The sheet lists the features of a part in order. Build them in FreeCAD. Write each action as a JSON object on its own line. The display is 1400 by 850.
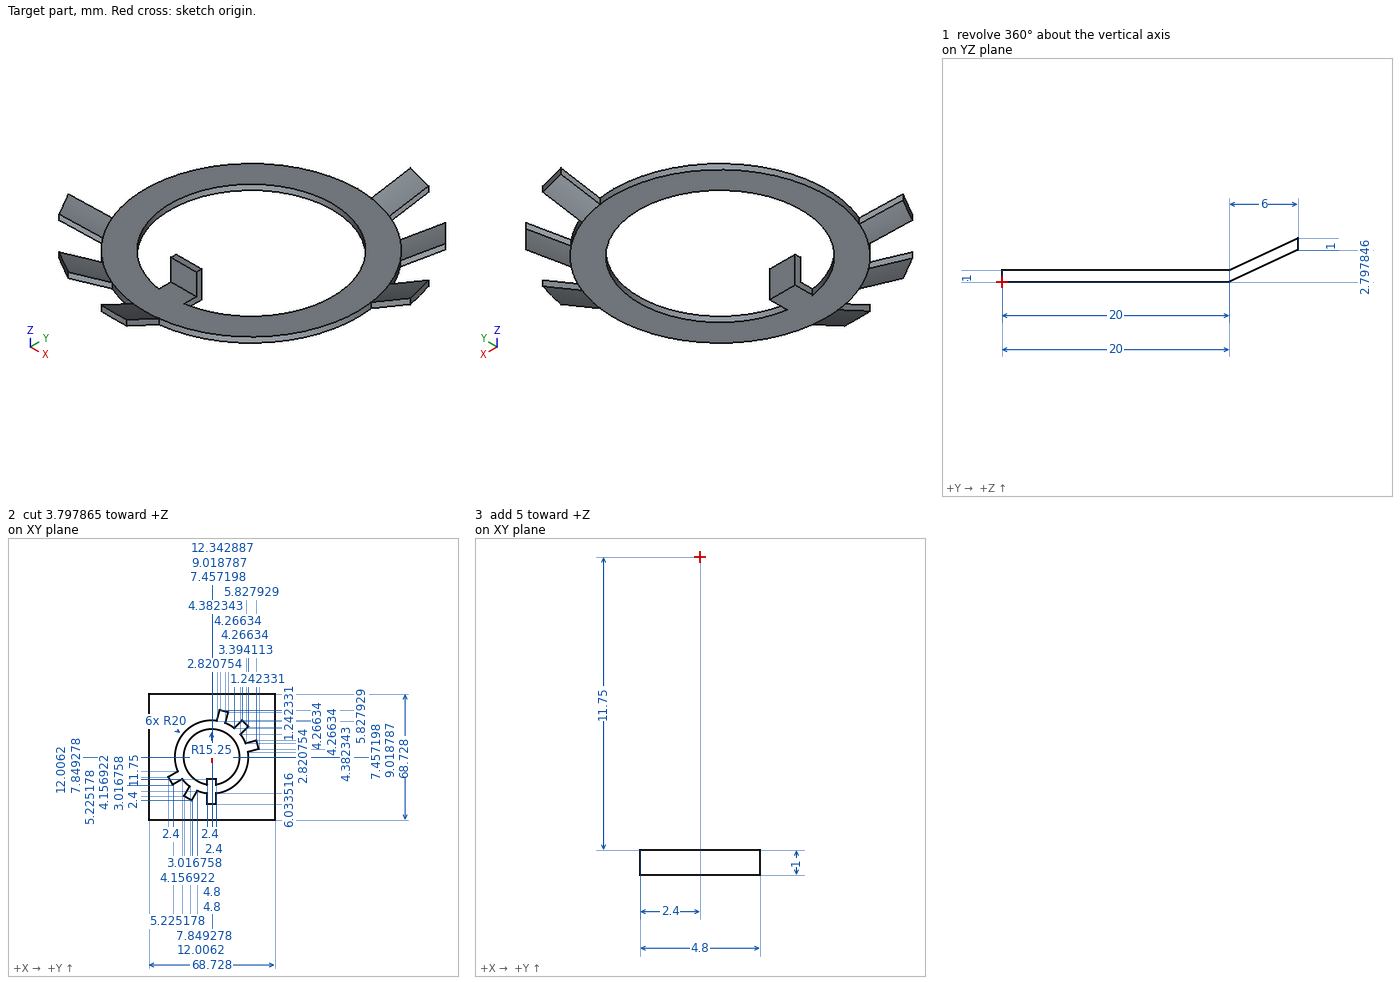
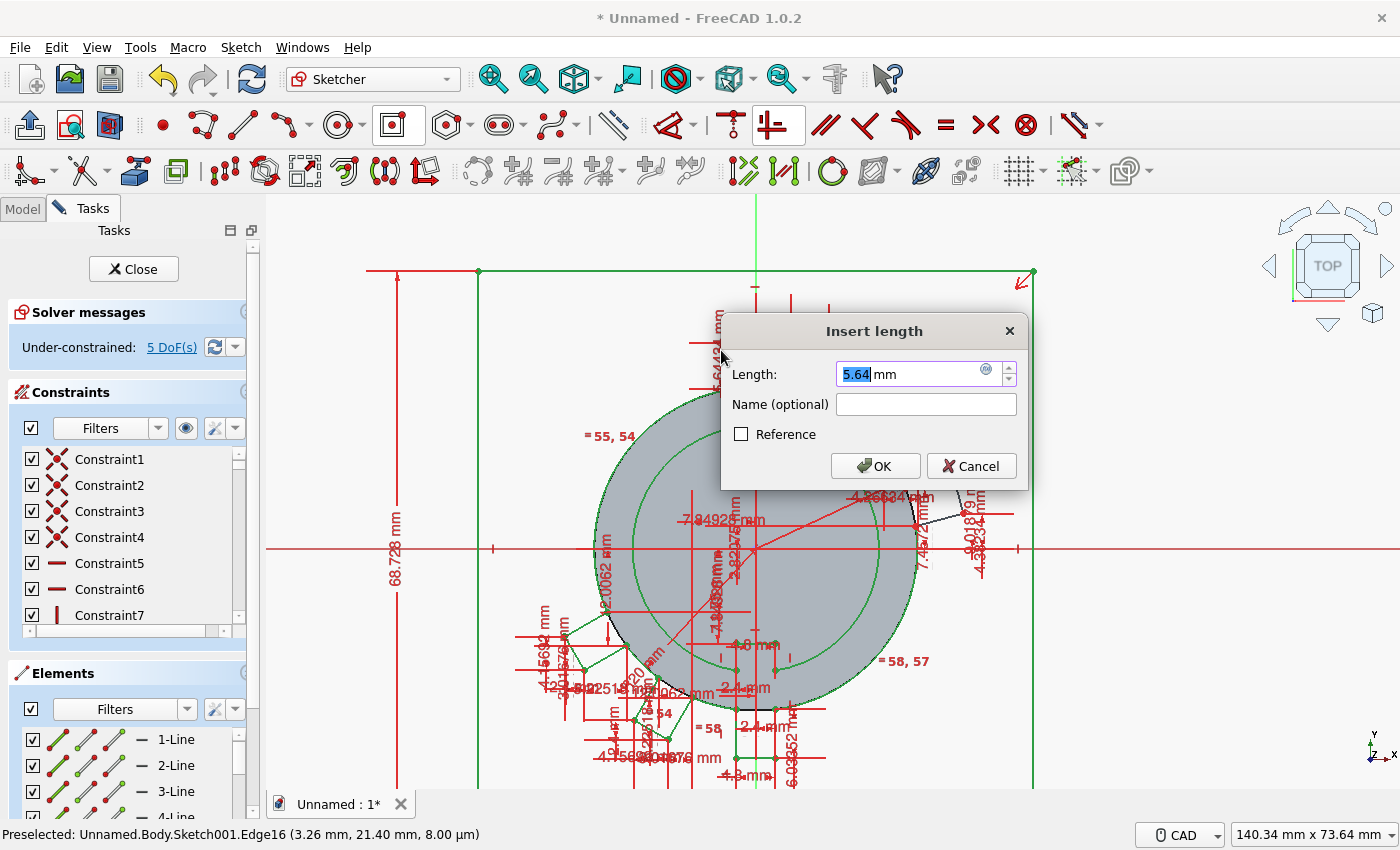
{"action": "type", "text": "5.827929"}
{"action": "key", "text": "Return"}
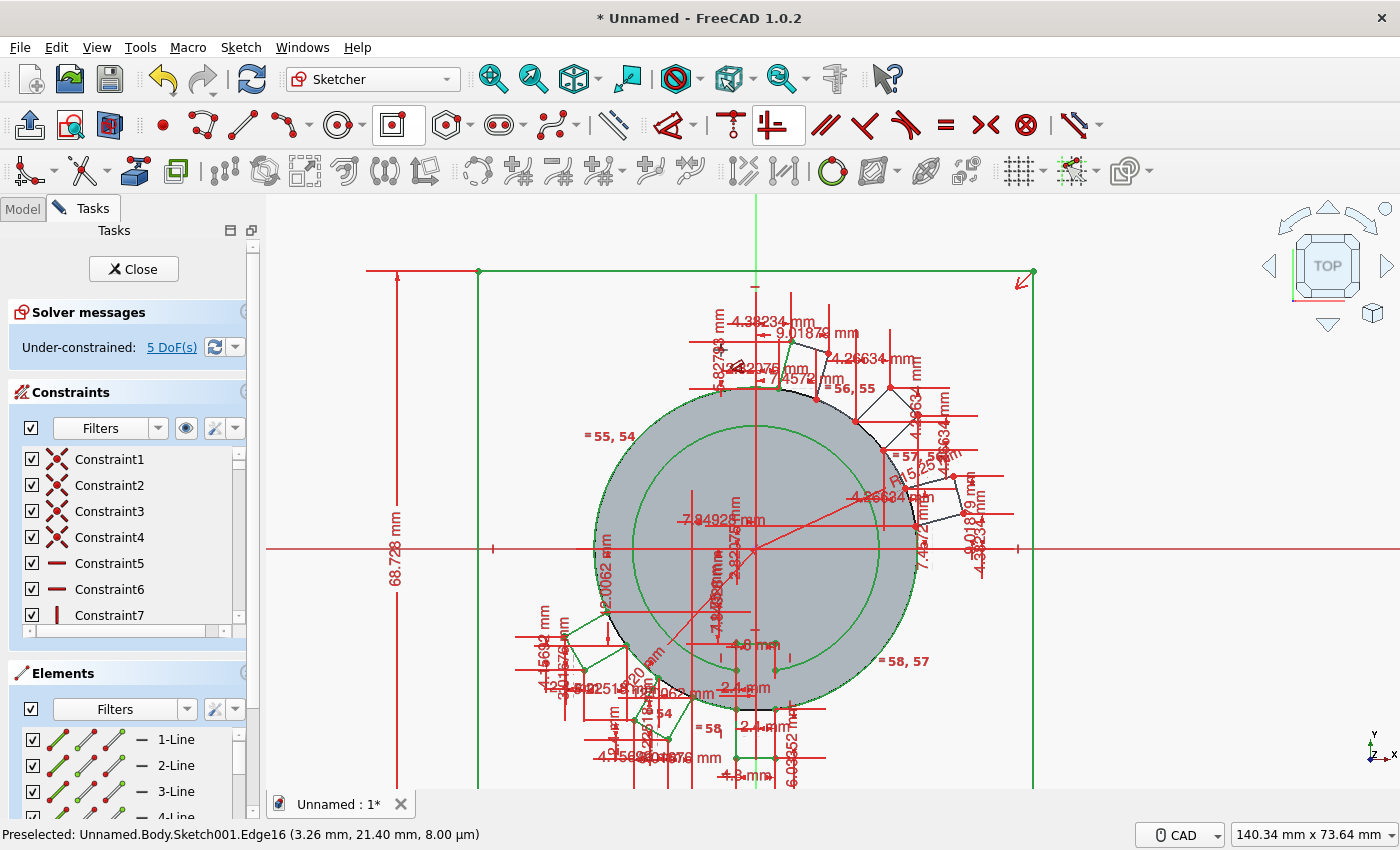
{"action": "scroll", "coordinate": [802, 345], "scroll_direction": "up", "scroll_amount": 7}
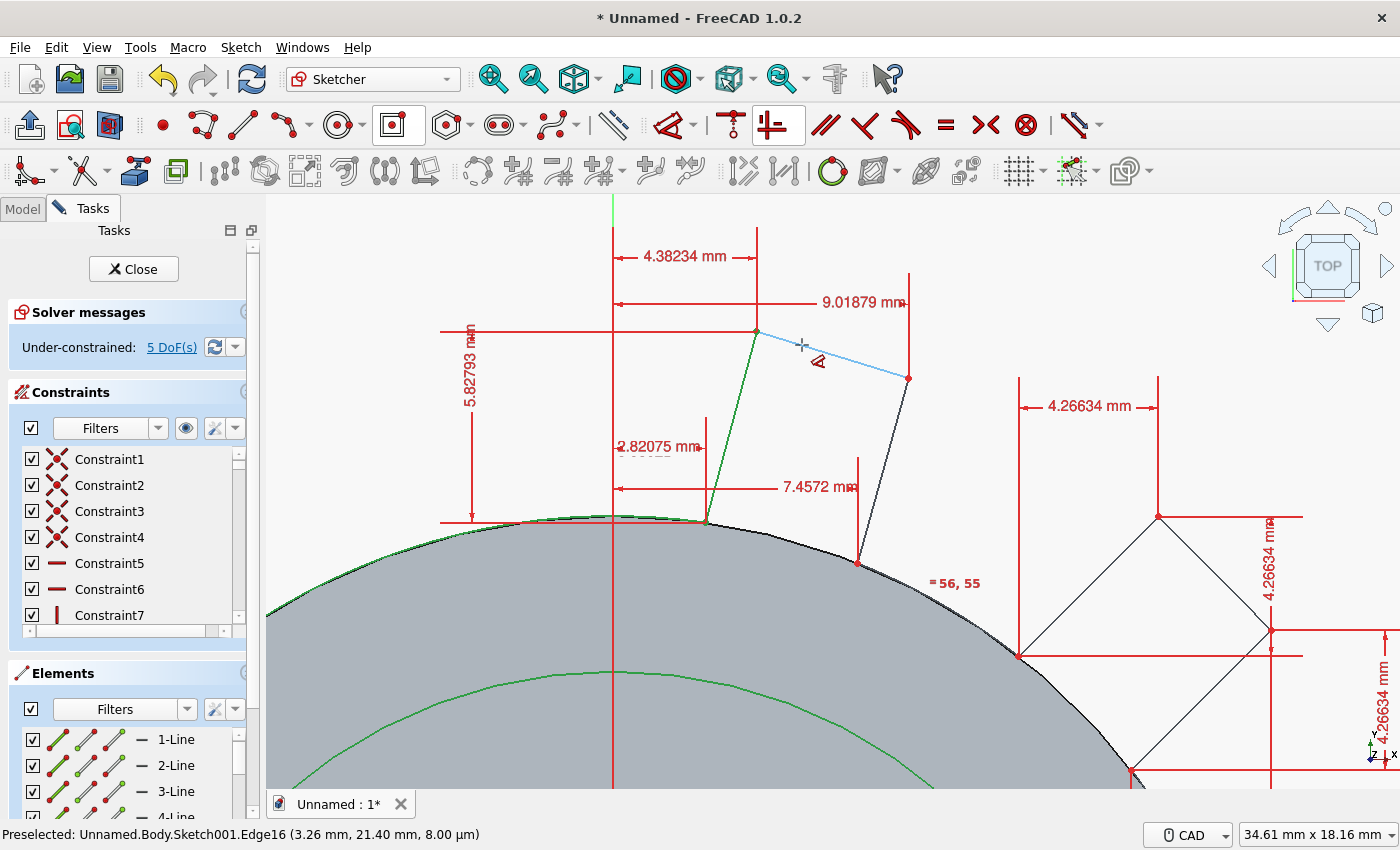
{"action": "left_click", "coordinate": [802, 346]}
{"action": "left_click", "coordinate": [943, 355]}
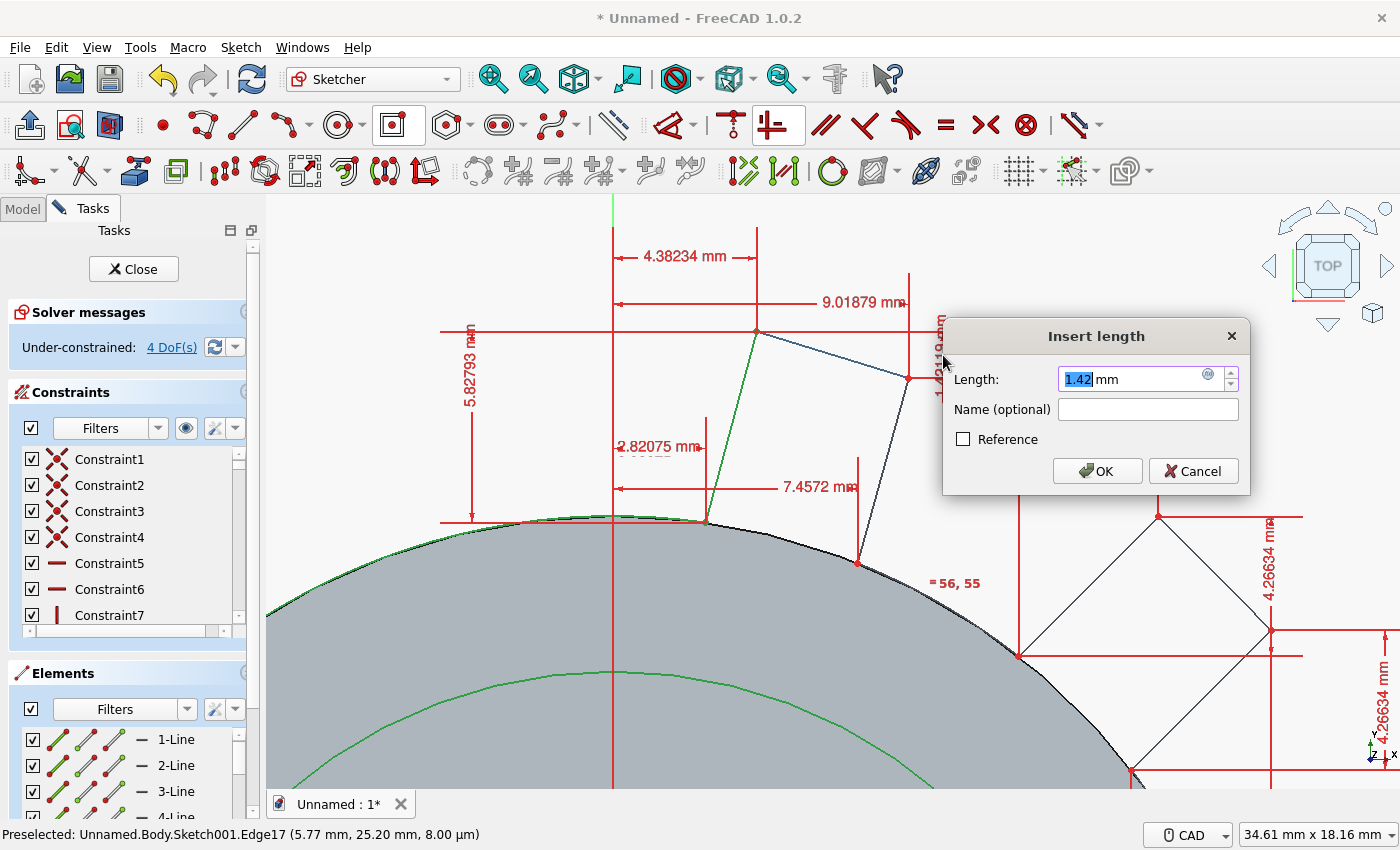
{"action": "type", "text": "1.242331"}
{"action": "key", "text": "Return"}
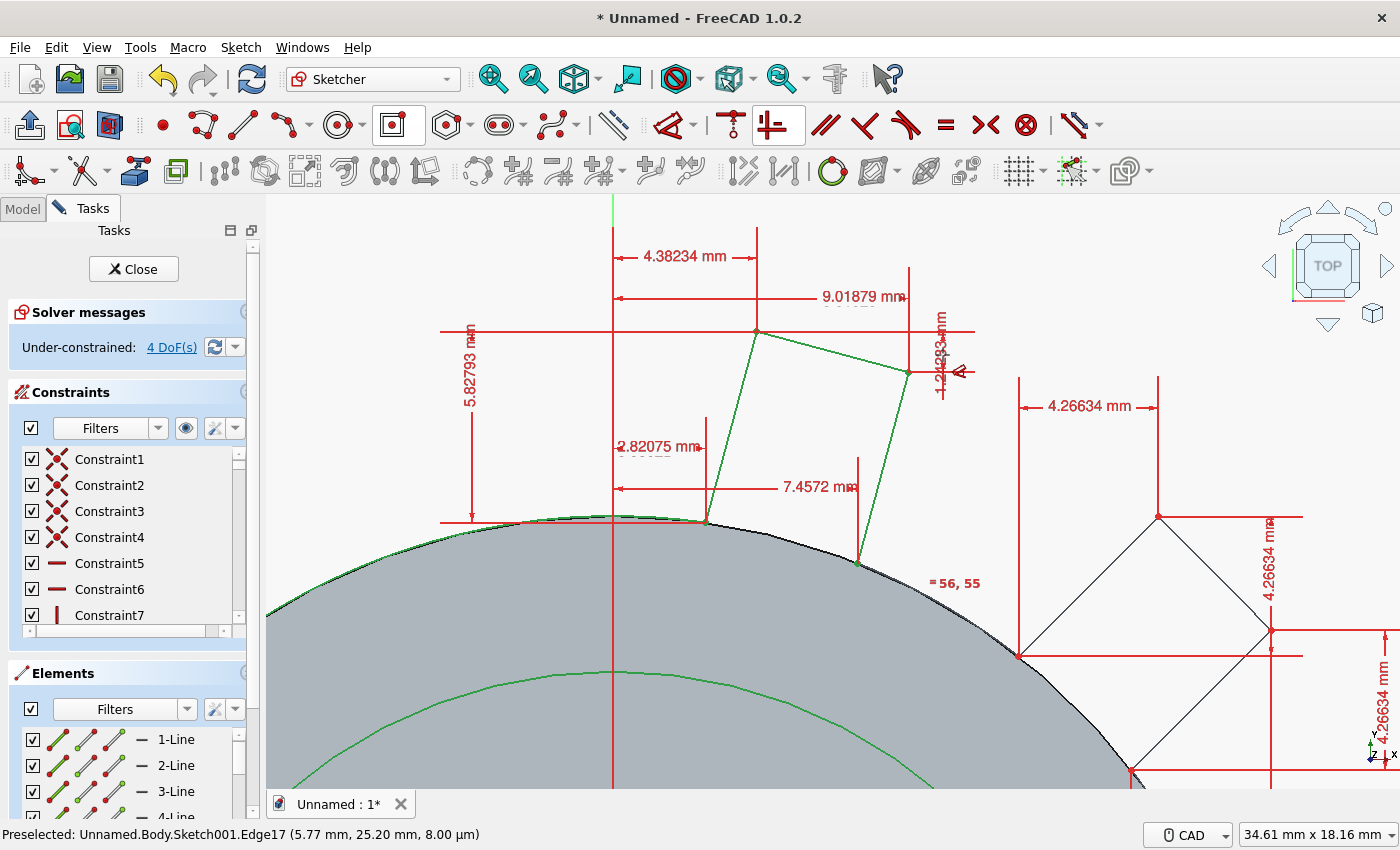
{"action": "left_click", "coordinate": [1192, 551]}
{"action": "left_click", "coordinate": [1197, 483]}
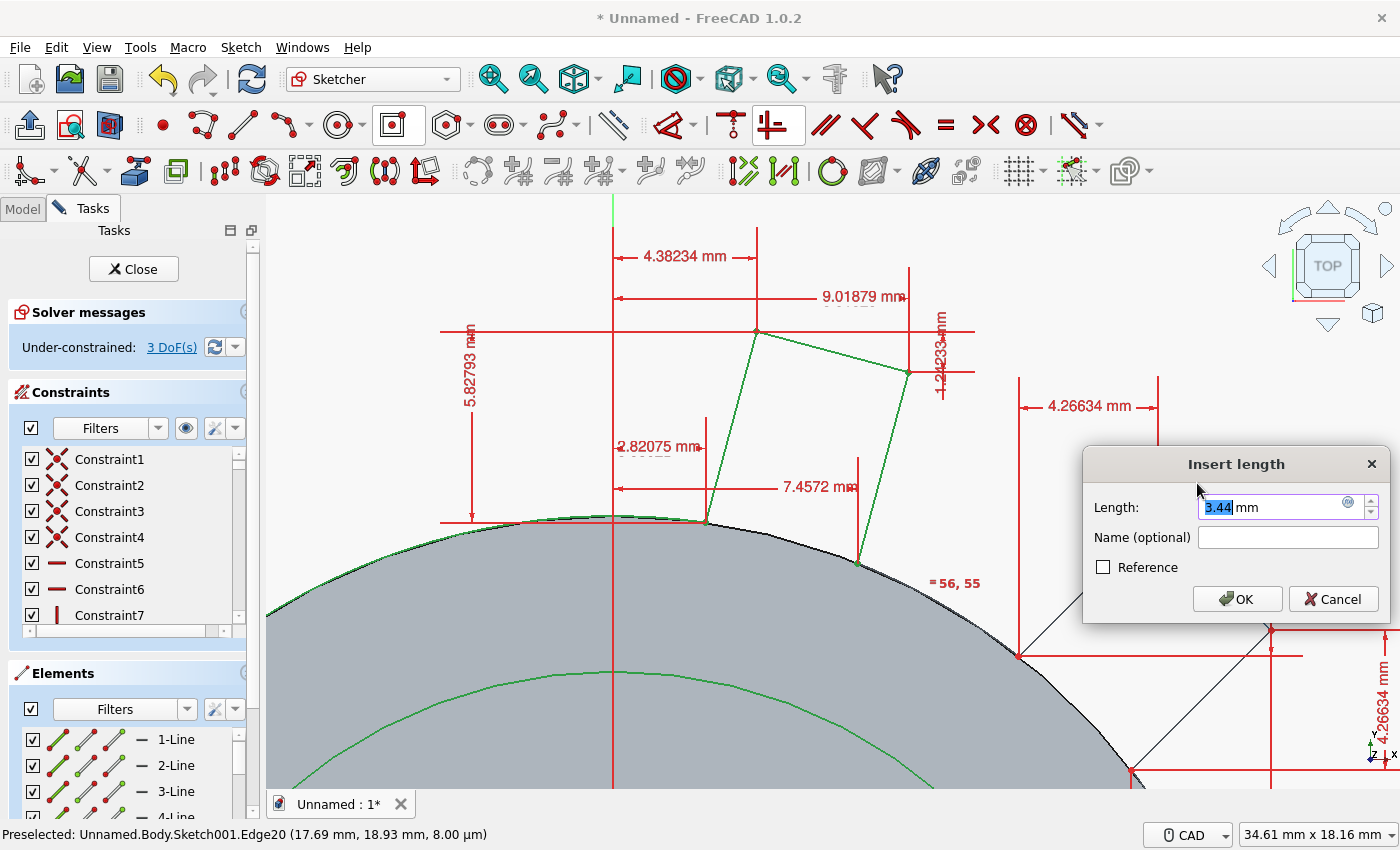
{"action": "type", "text": "3.394113"}
{"action": "key", "text": "Return"}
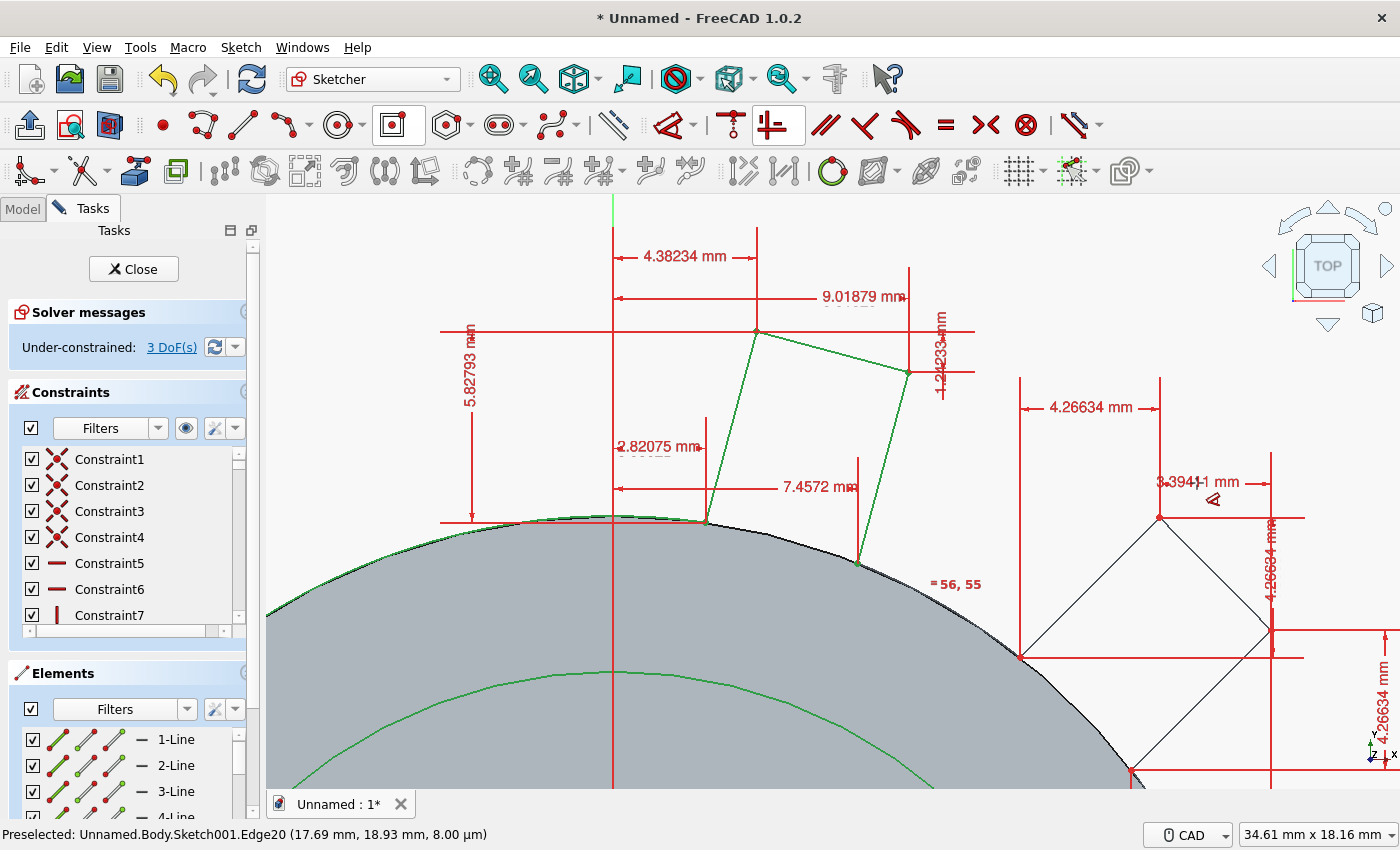
{"action": "scroll", "coordinate": [794, 357], "scroll_direction": "down", "scroll_amount": 9}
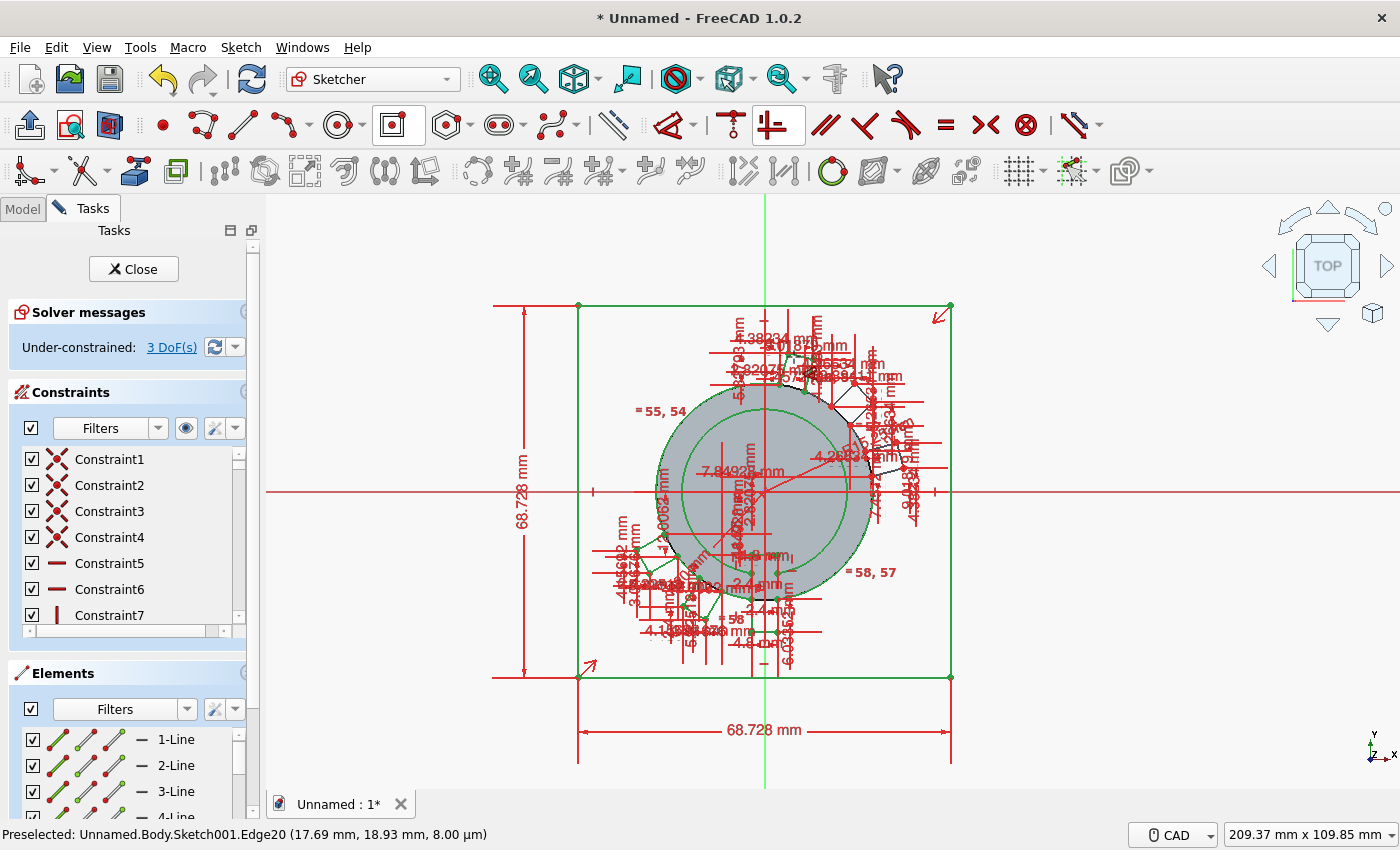
{"action": "scroll", "coordinate": [875, 449], "scroll_direction": "up", "scroll_amount": 2}